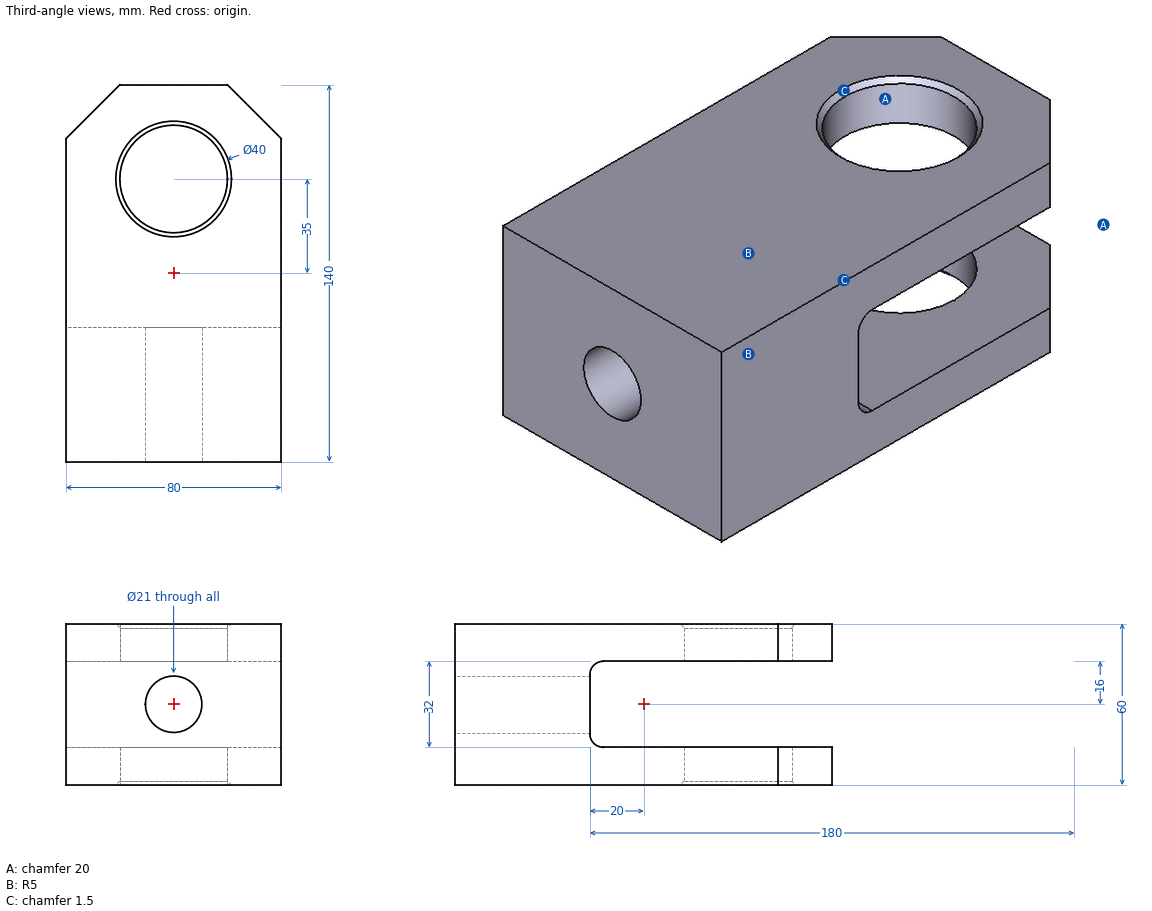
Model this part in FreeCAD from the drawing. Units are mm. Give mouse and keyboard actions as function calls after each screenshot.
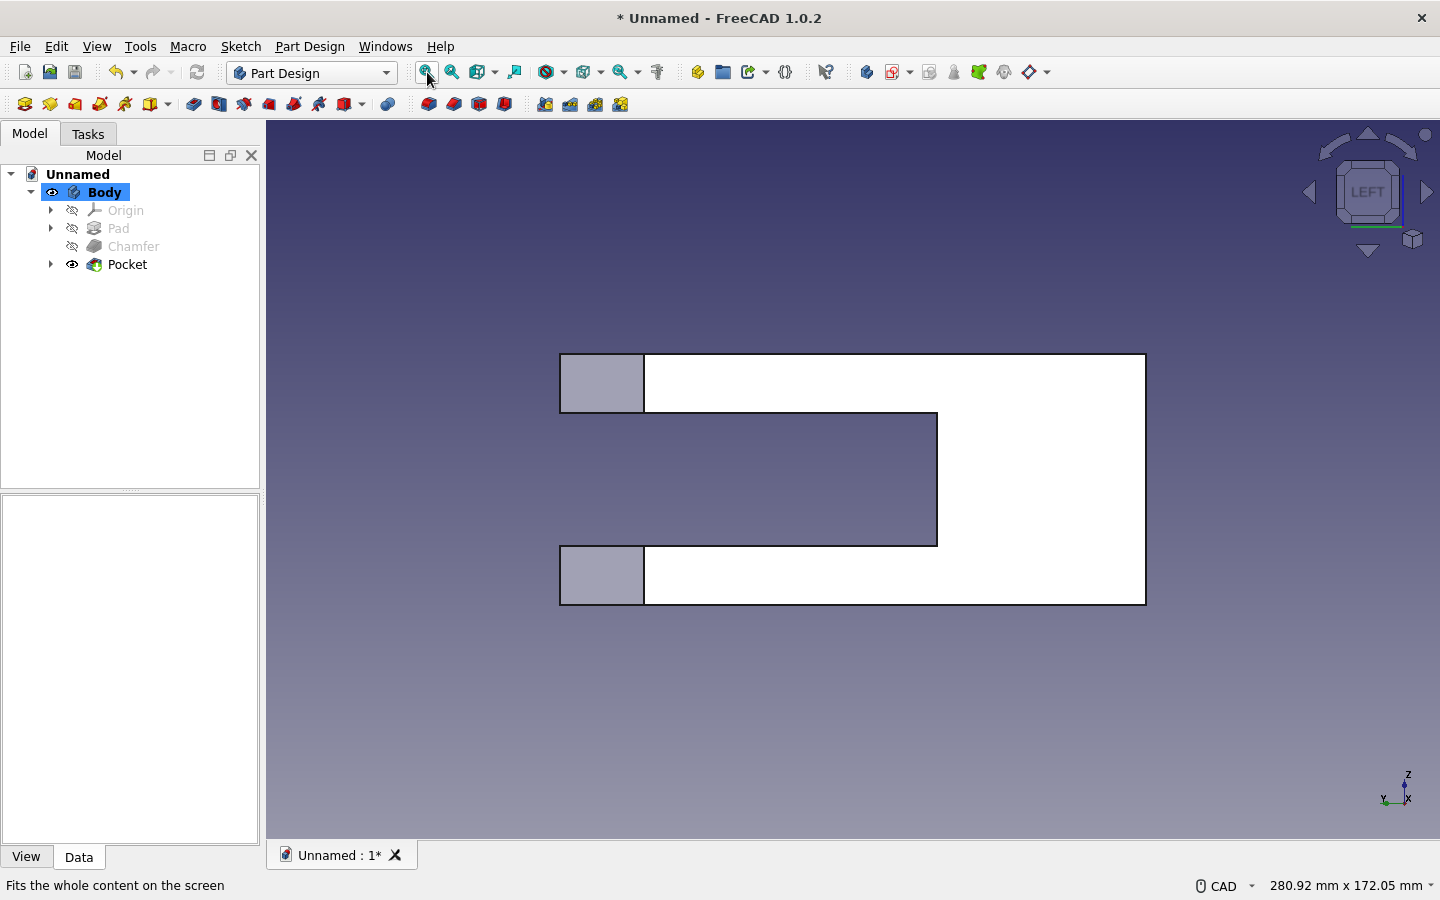
key(v)
key(3)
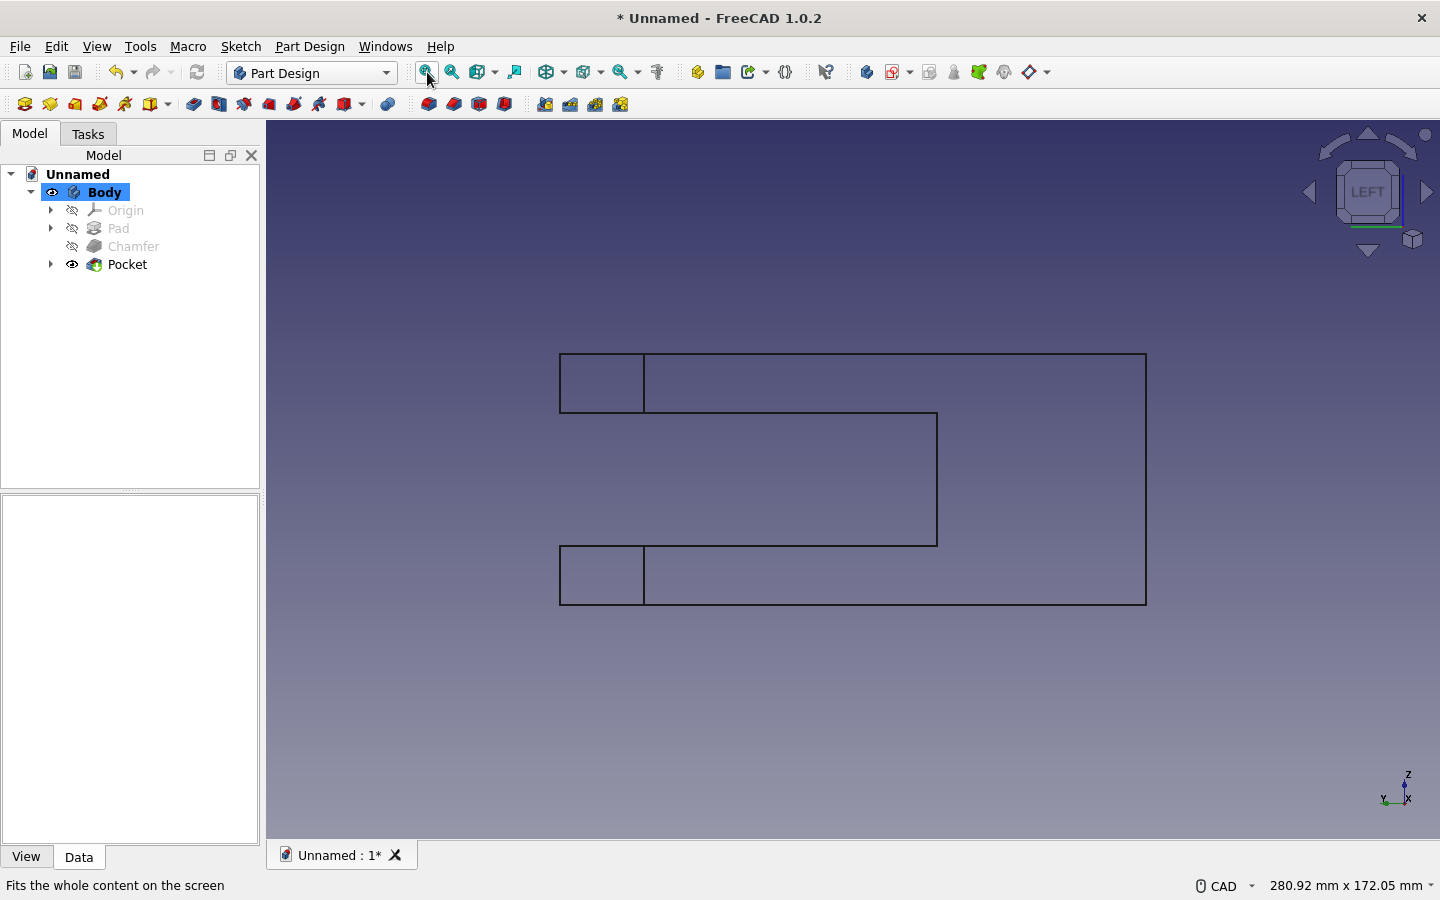
key(0)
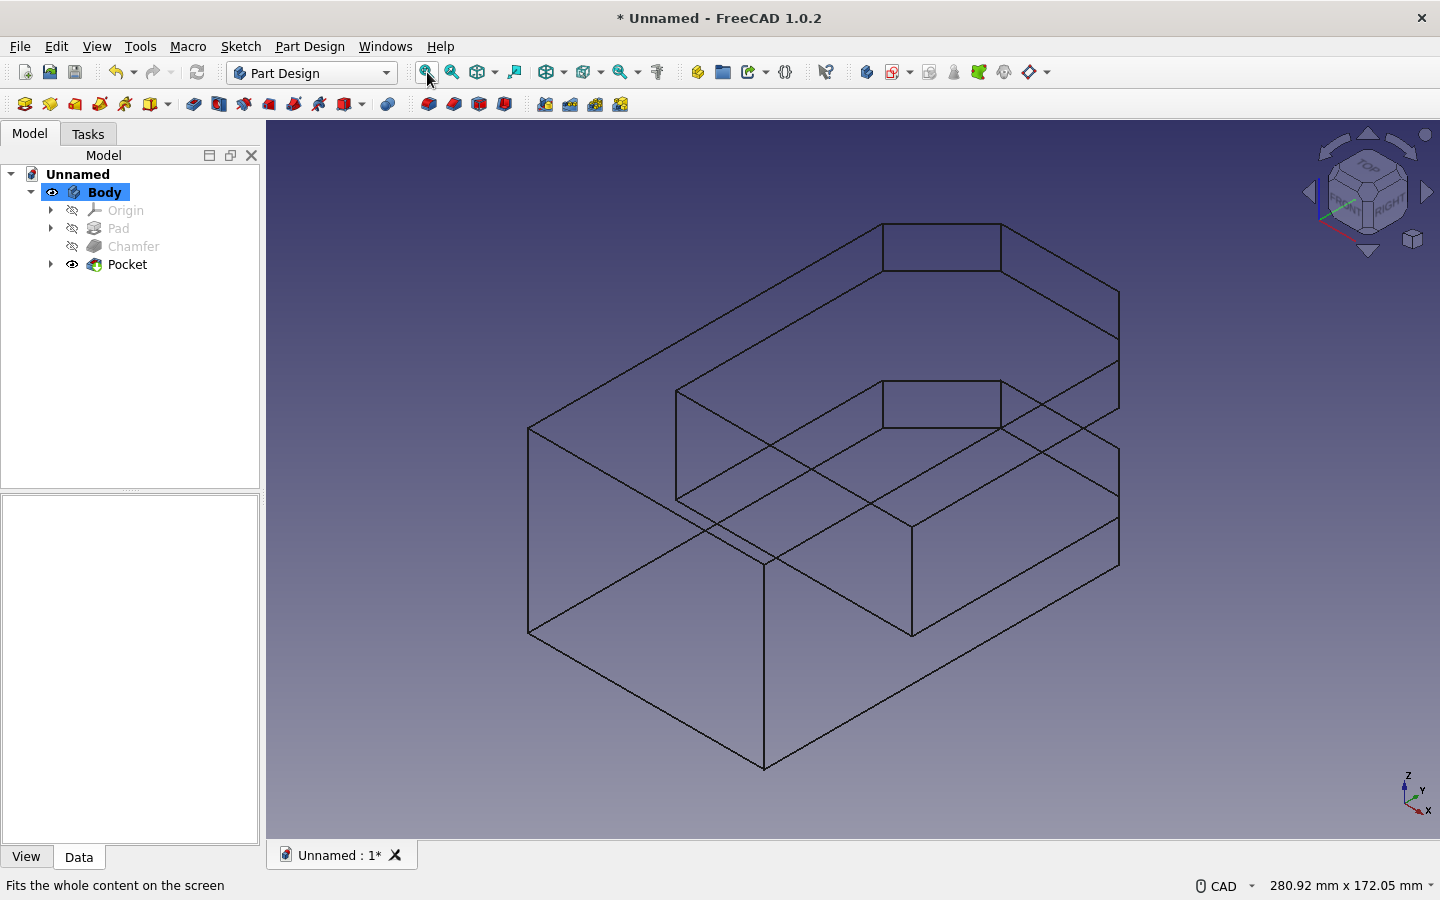
click(794, 458)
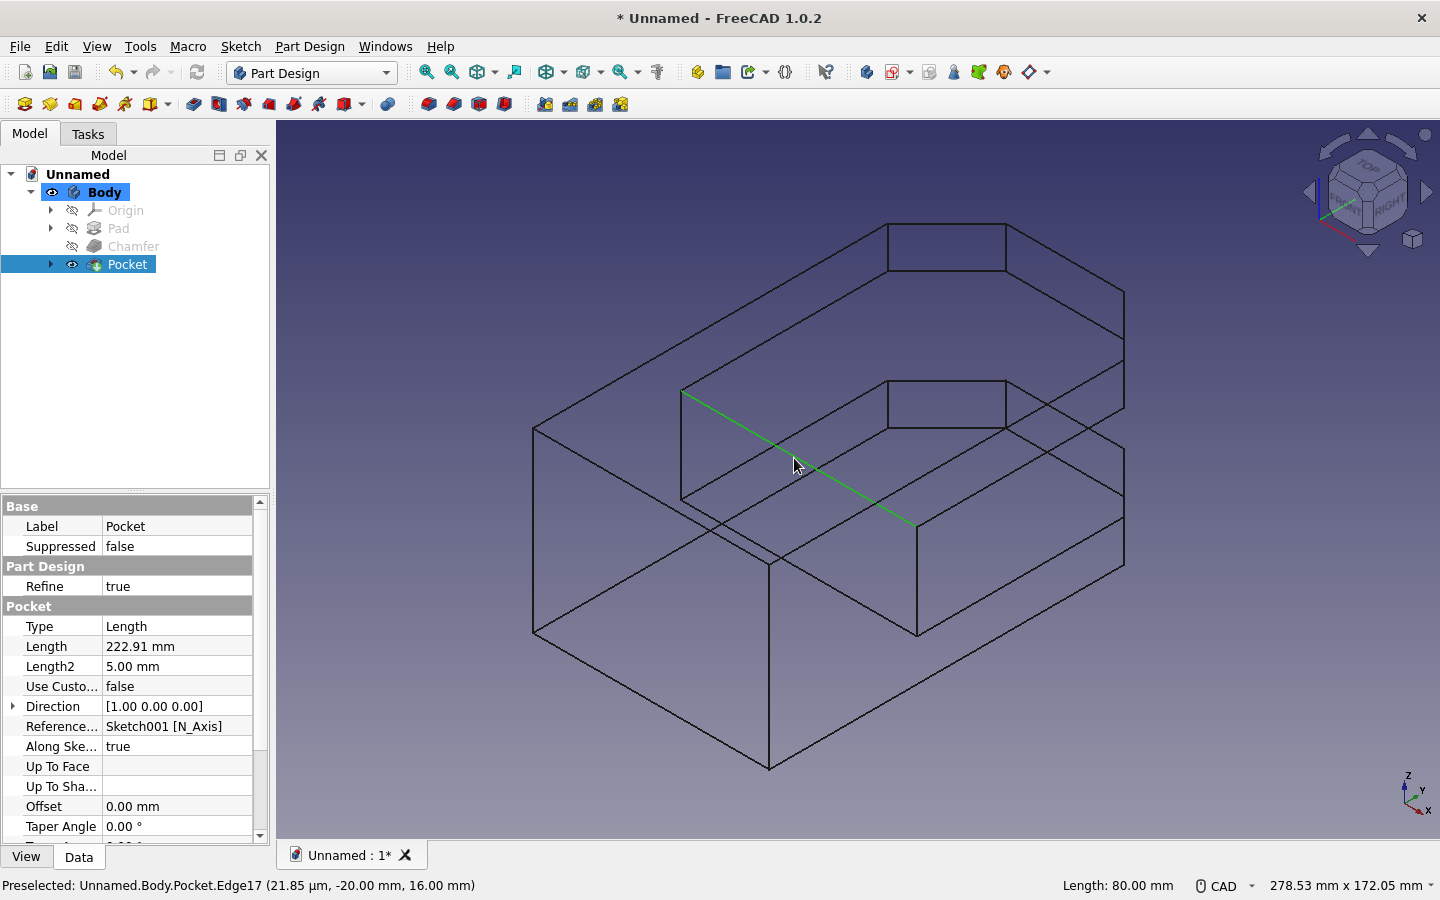
click(799, 567, ctrl)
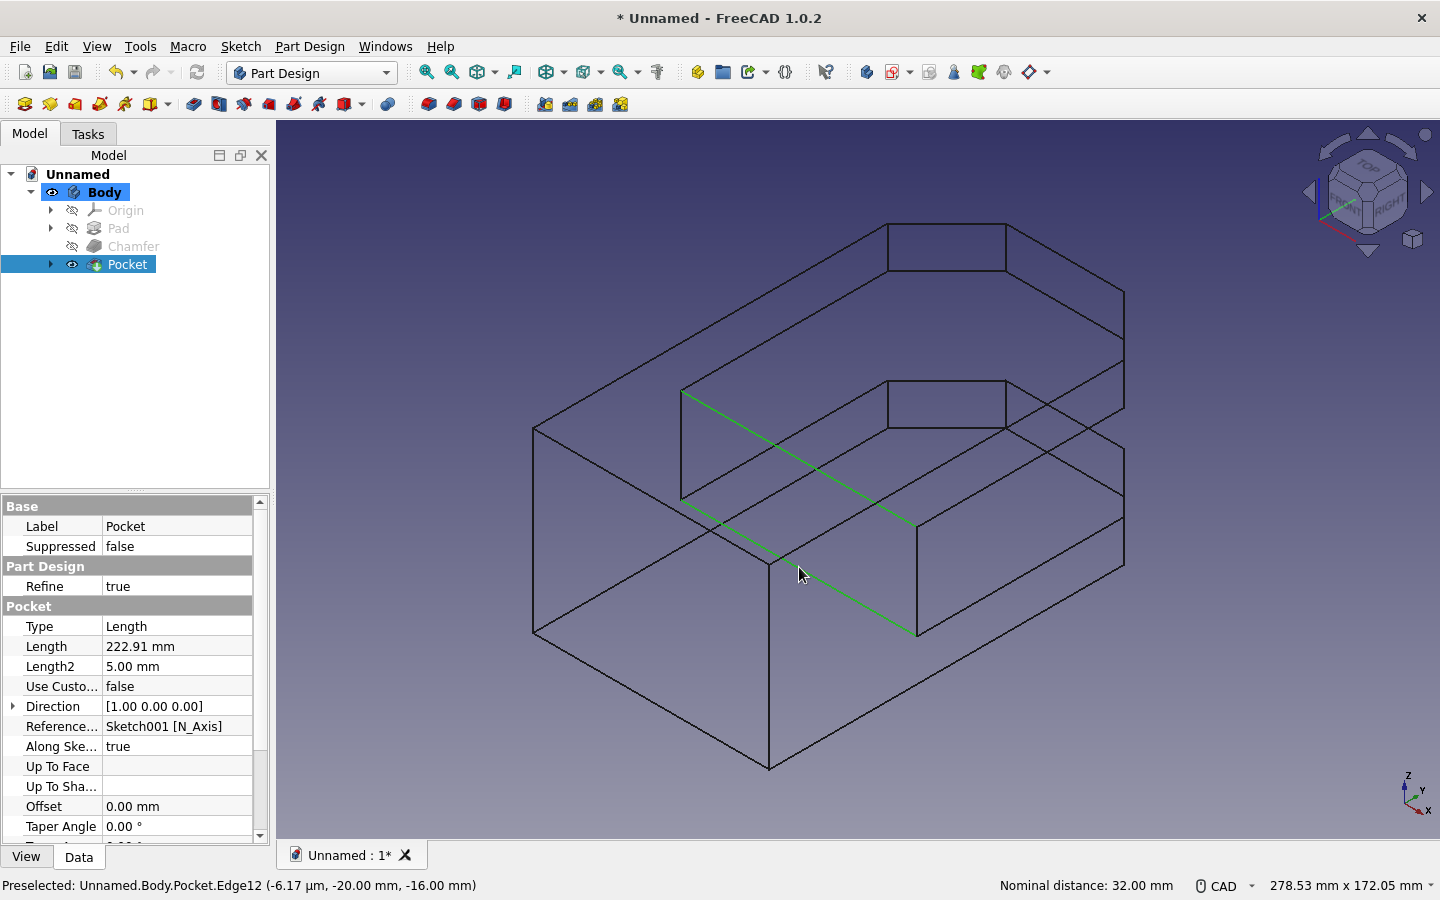
key(v)
key(1)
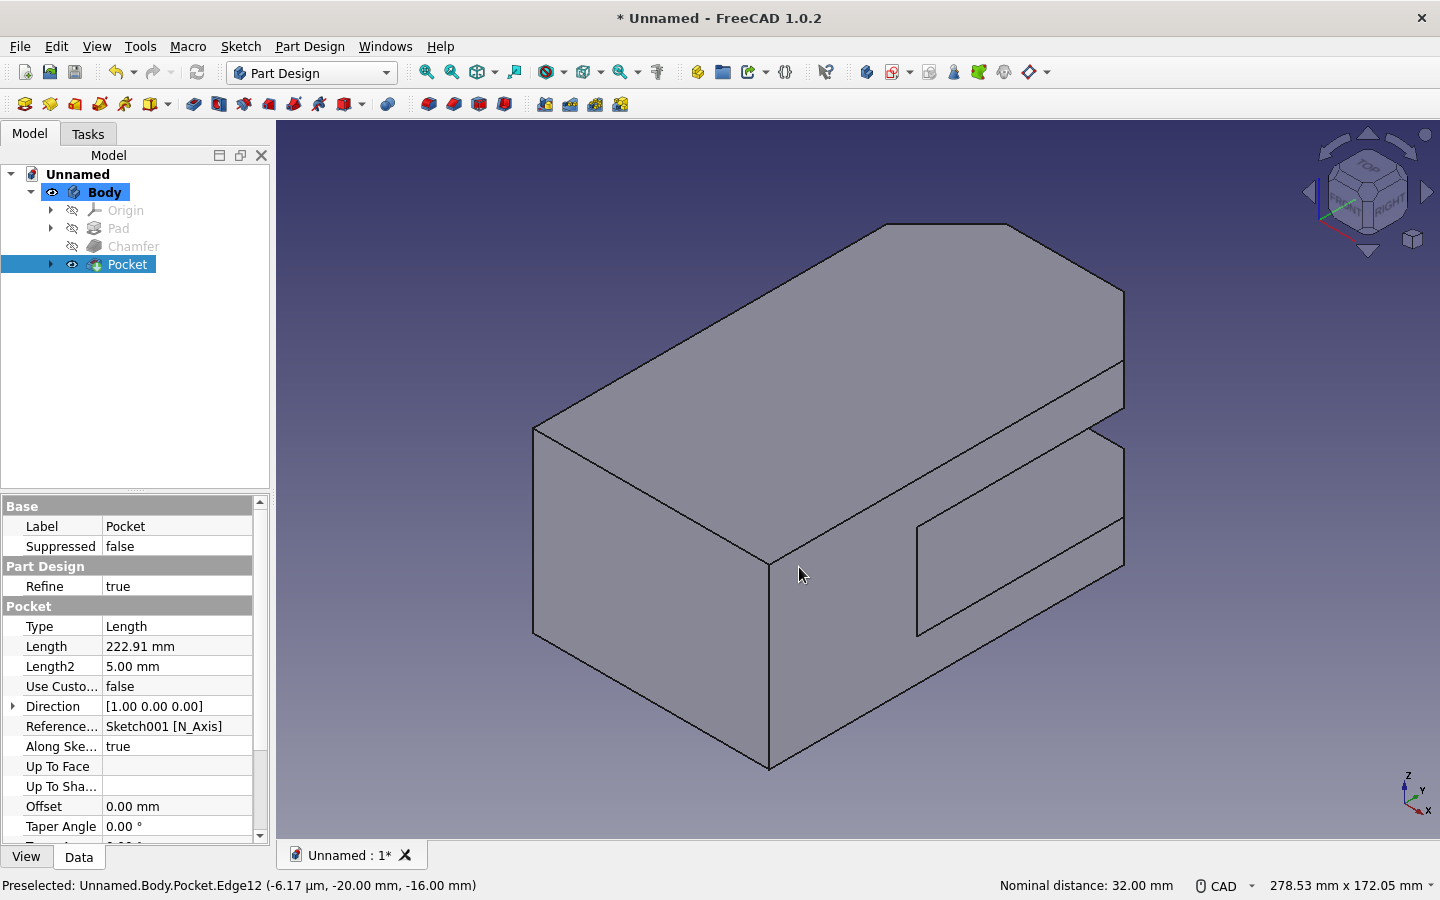
click(429, 104)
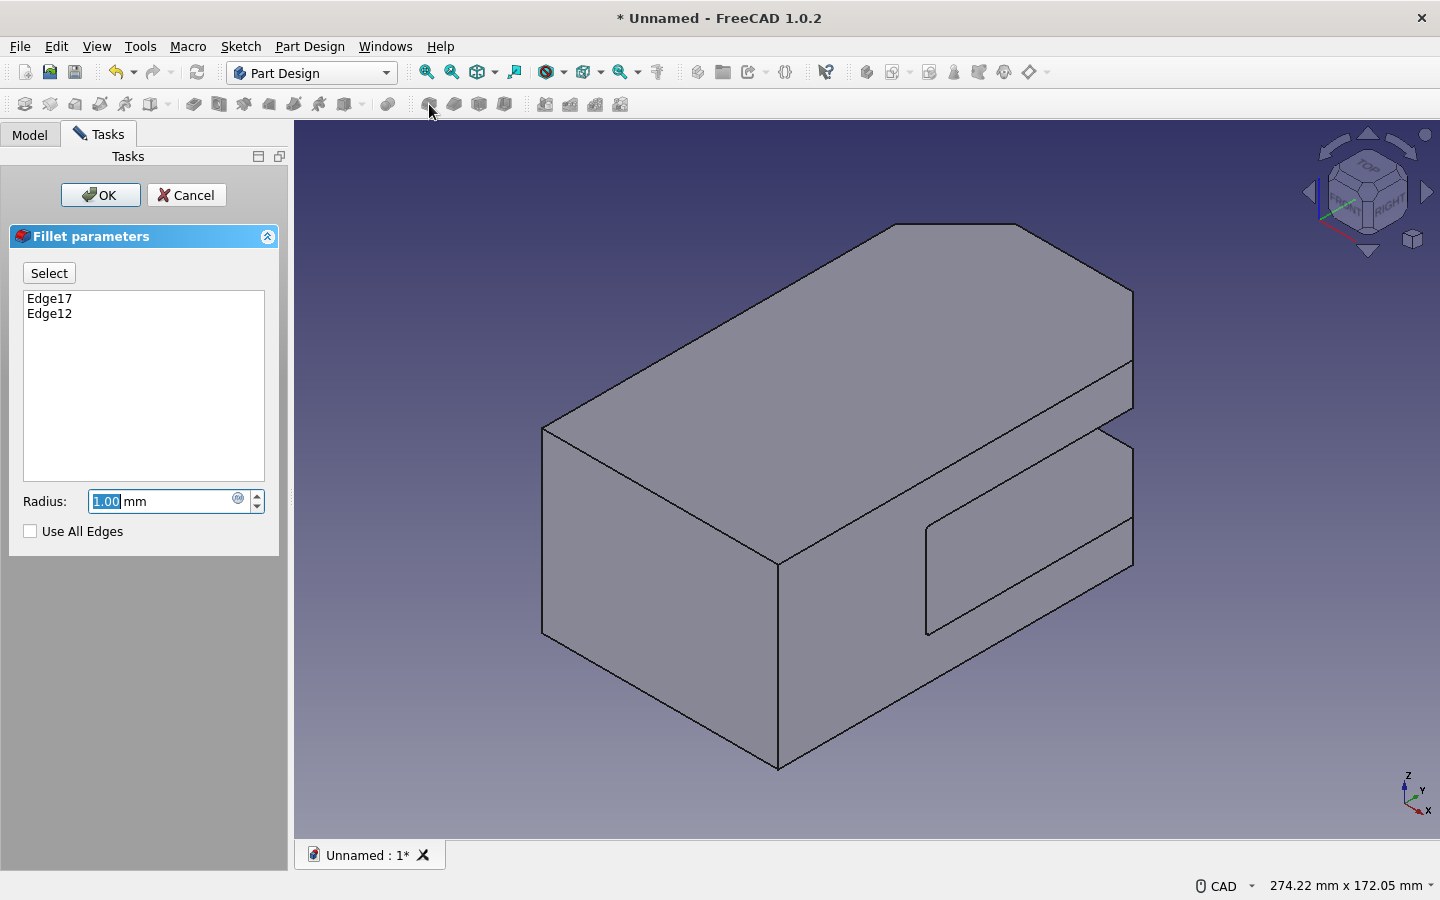
text(5)
key(Tab)